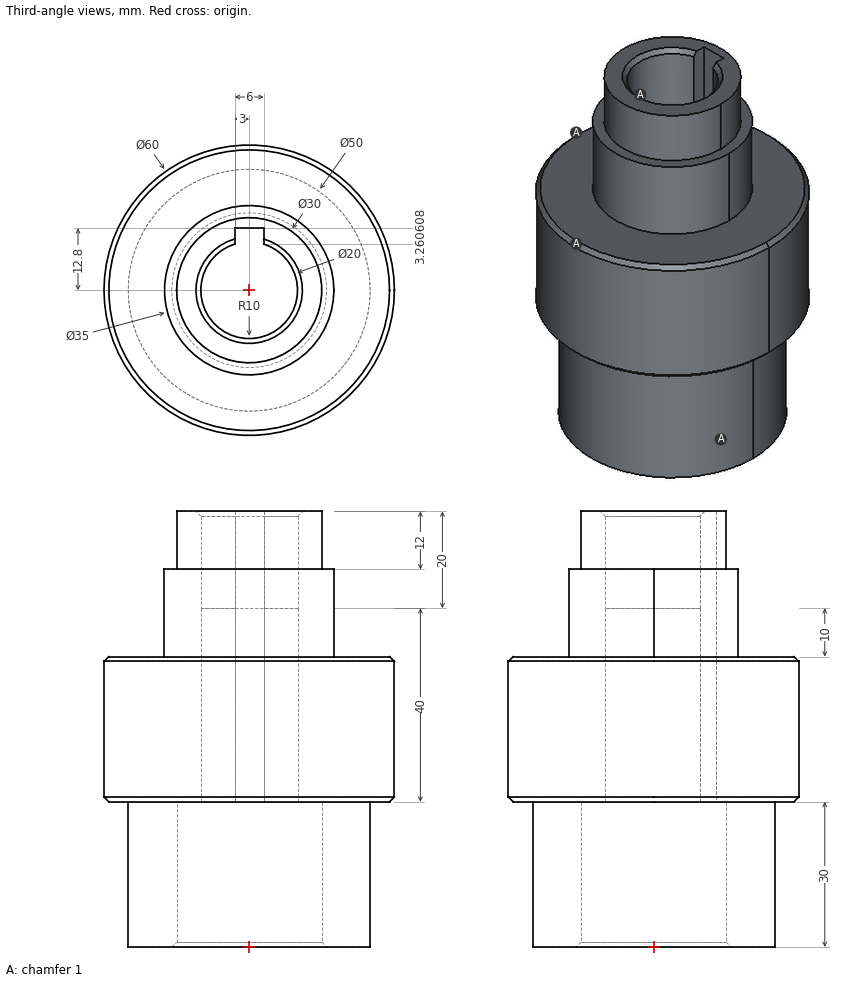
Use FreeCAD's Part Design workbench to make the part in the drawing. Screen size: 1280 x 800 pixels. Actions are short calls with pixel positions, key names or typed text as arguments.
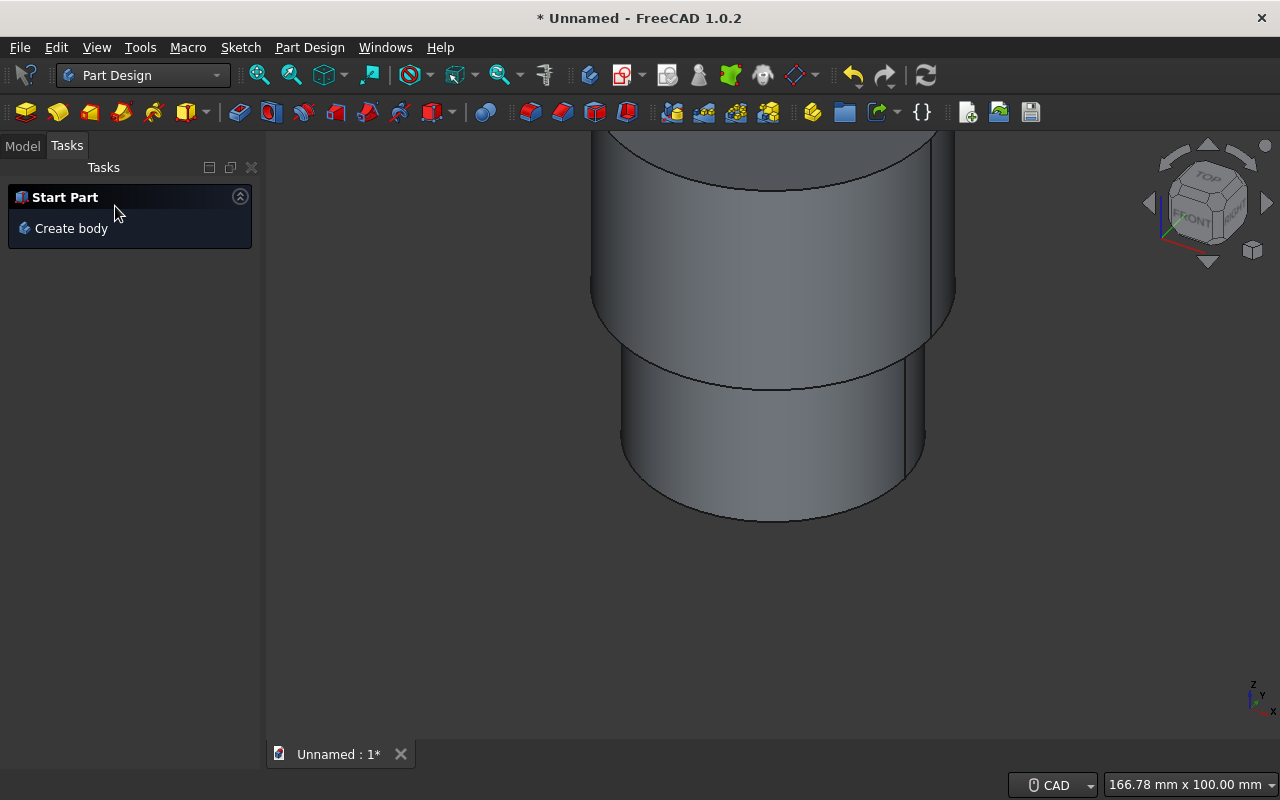
key(v)
key(f)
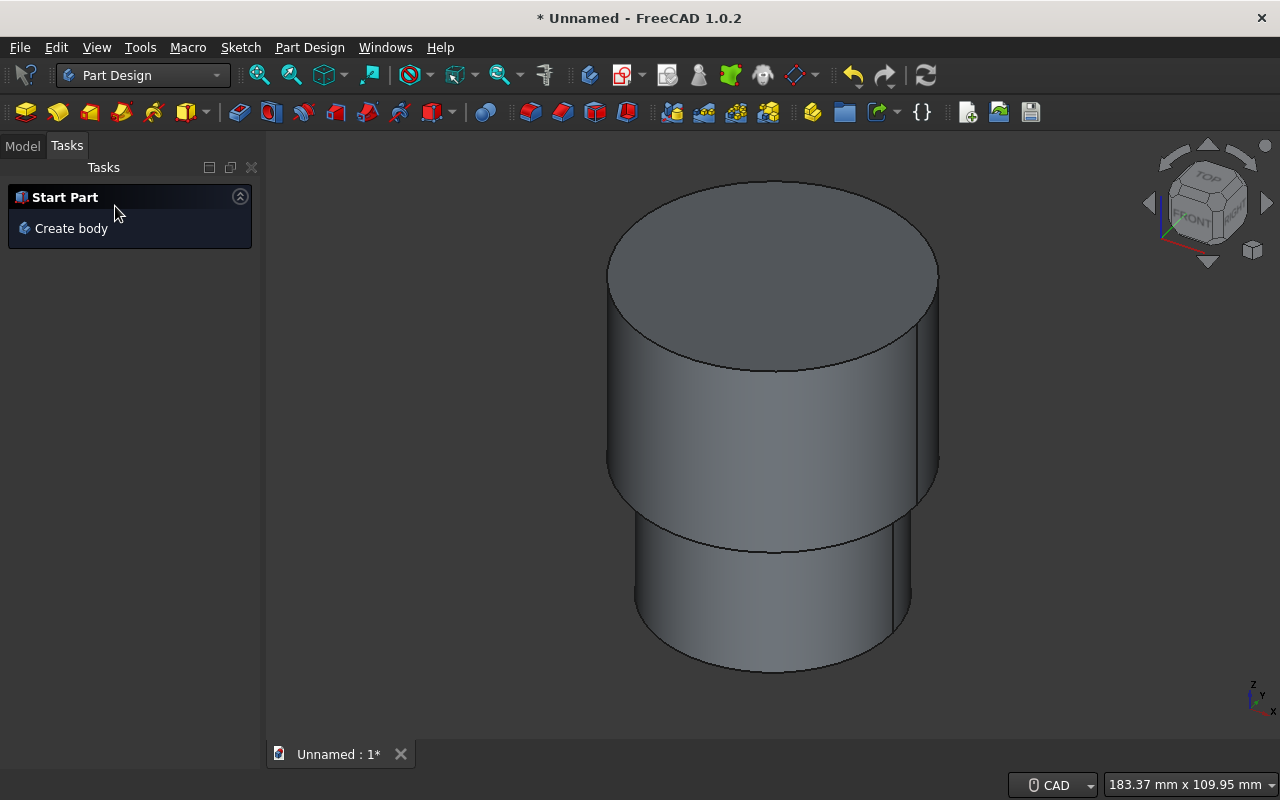
key(5)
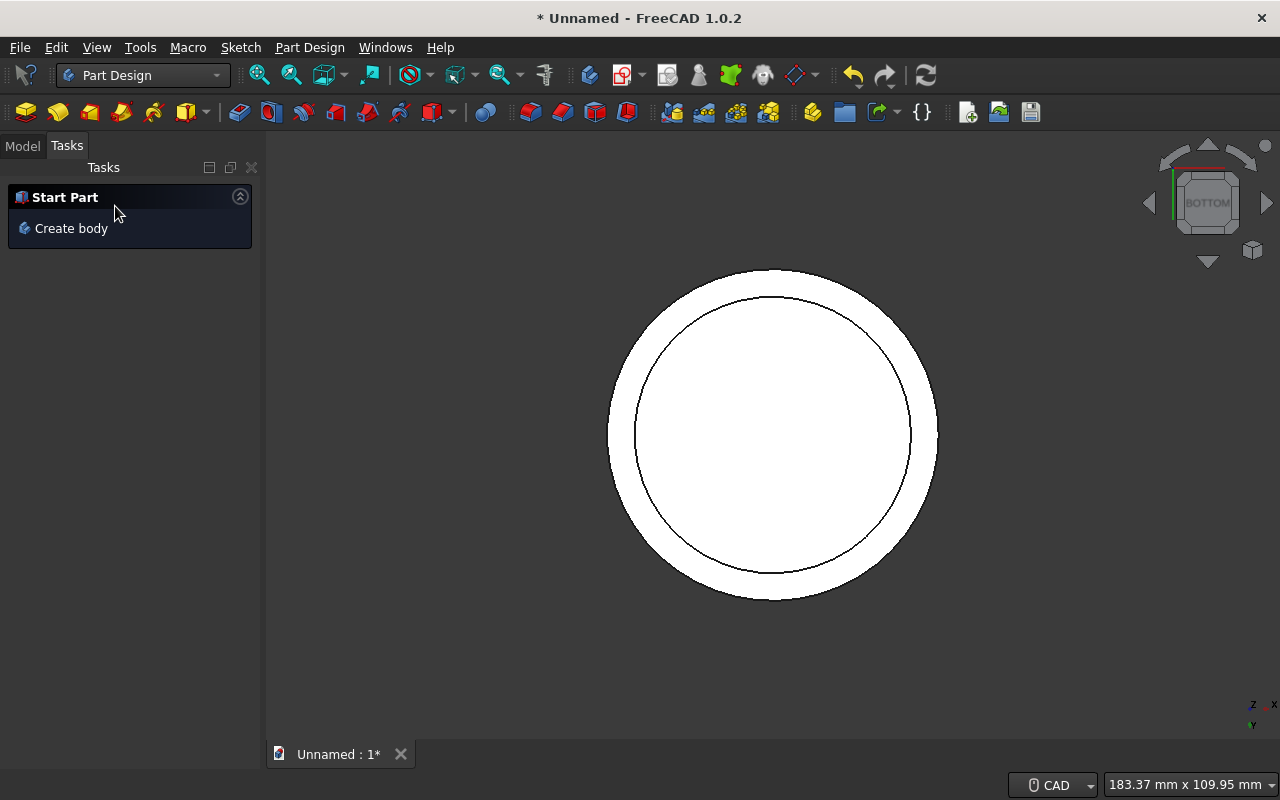
click(773, 434)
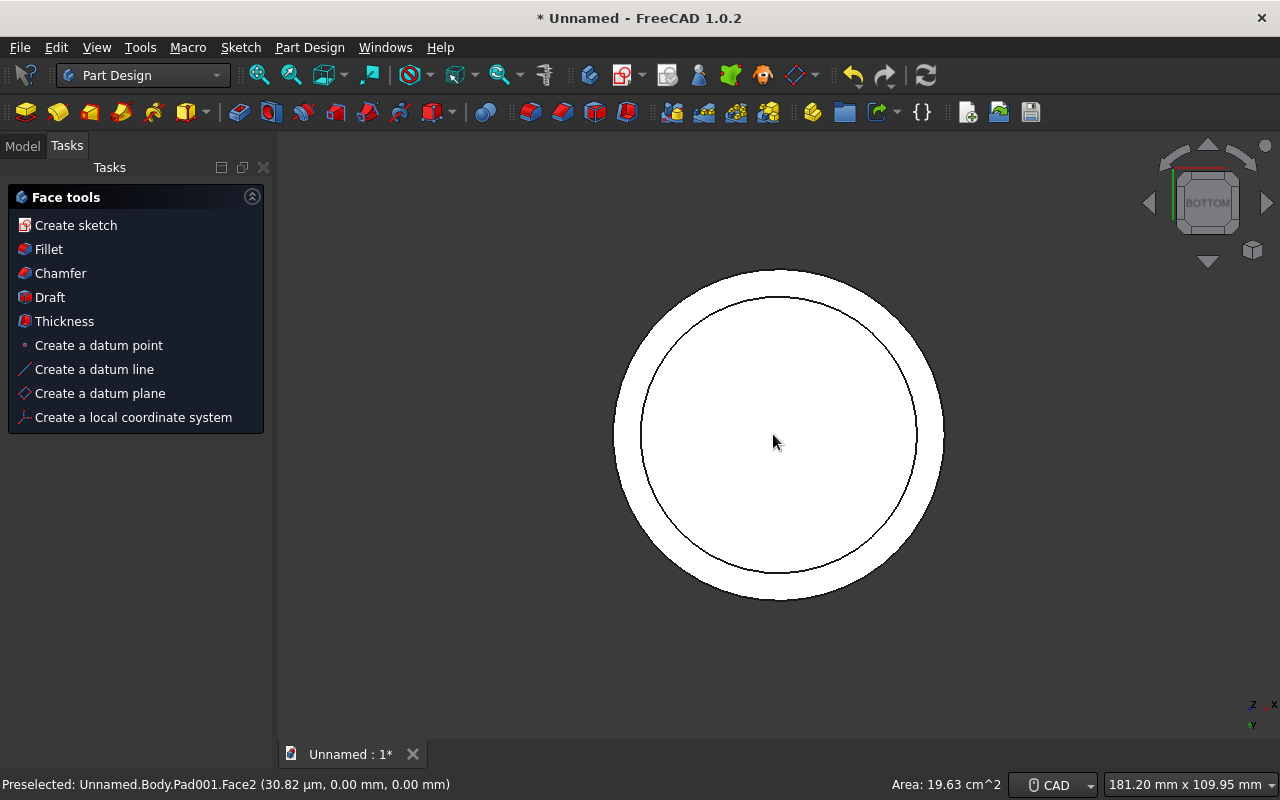
click(622, 76)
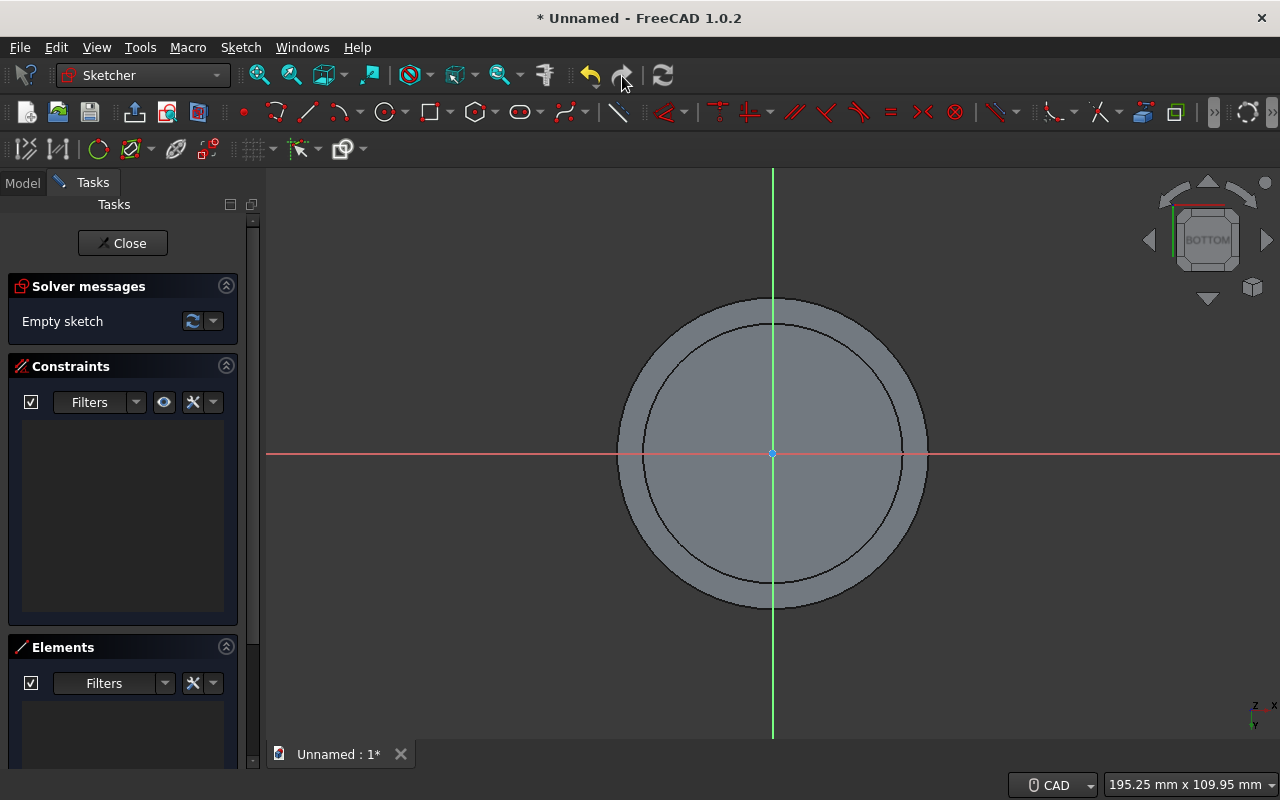
scroll(802, 454, up, 6)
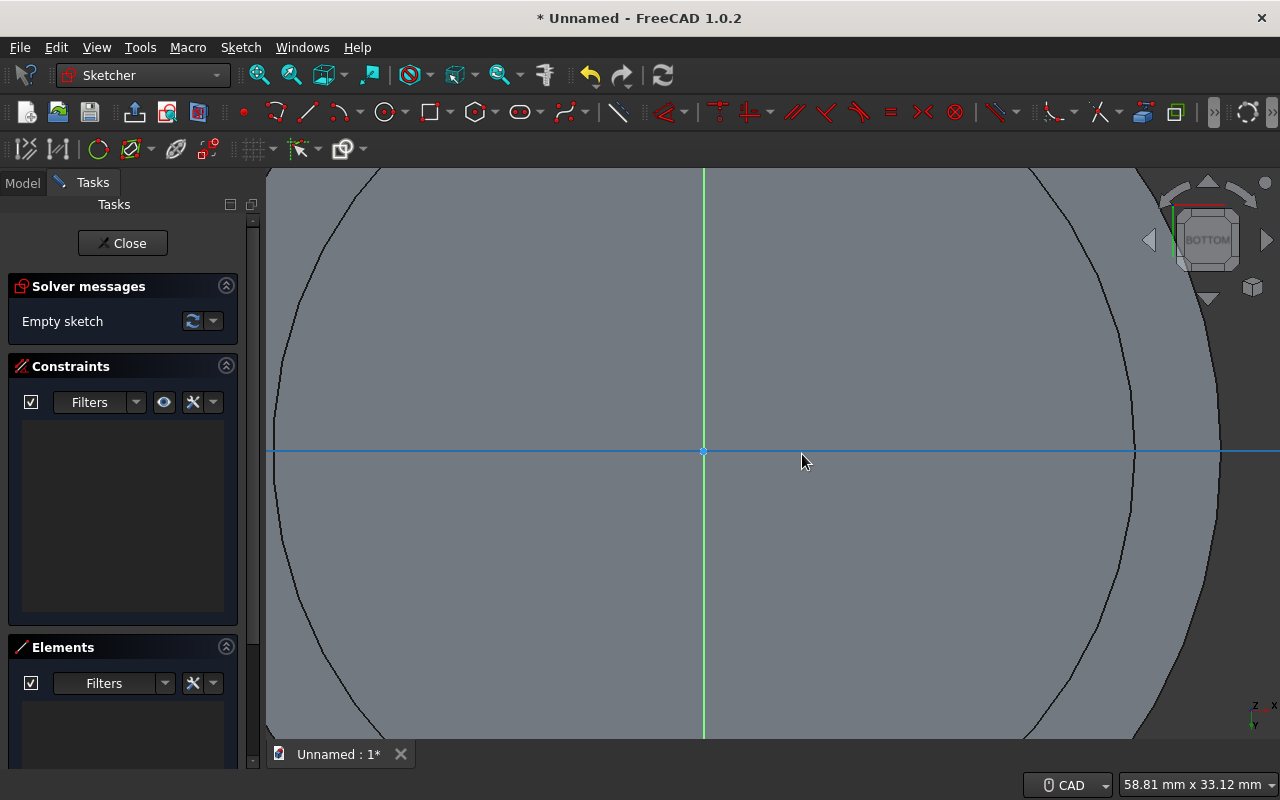
click(386, 112)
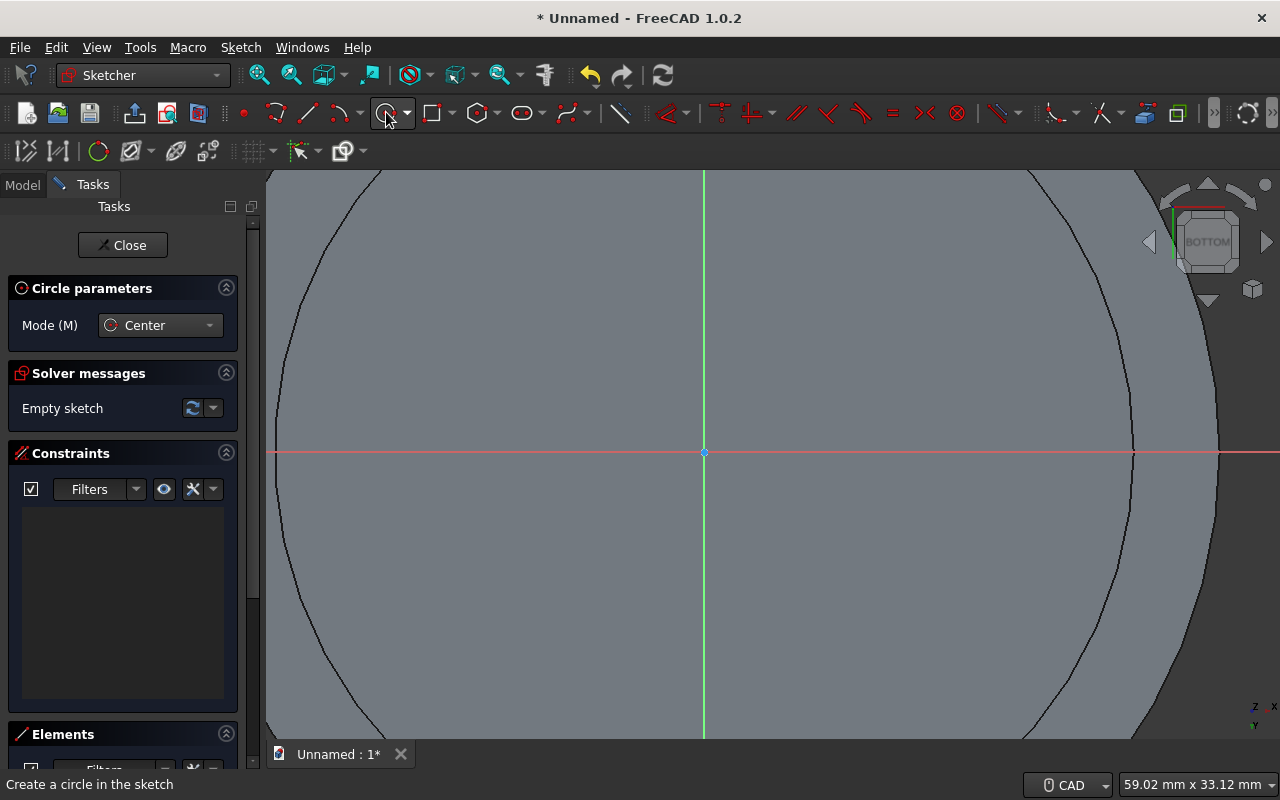
click(704, 452)
move(826, 331)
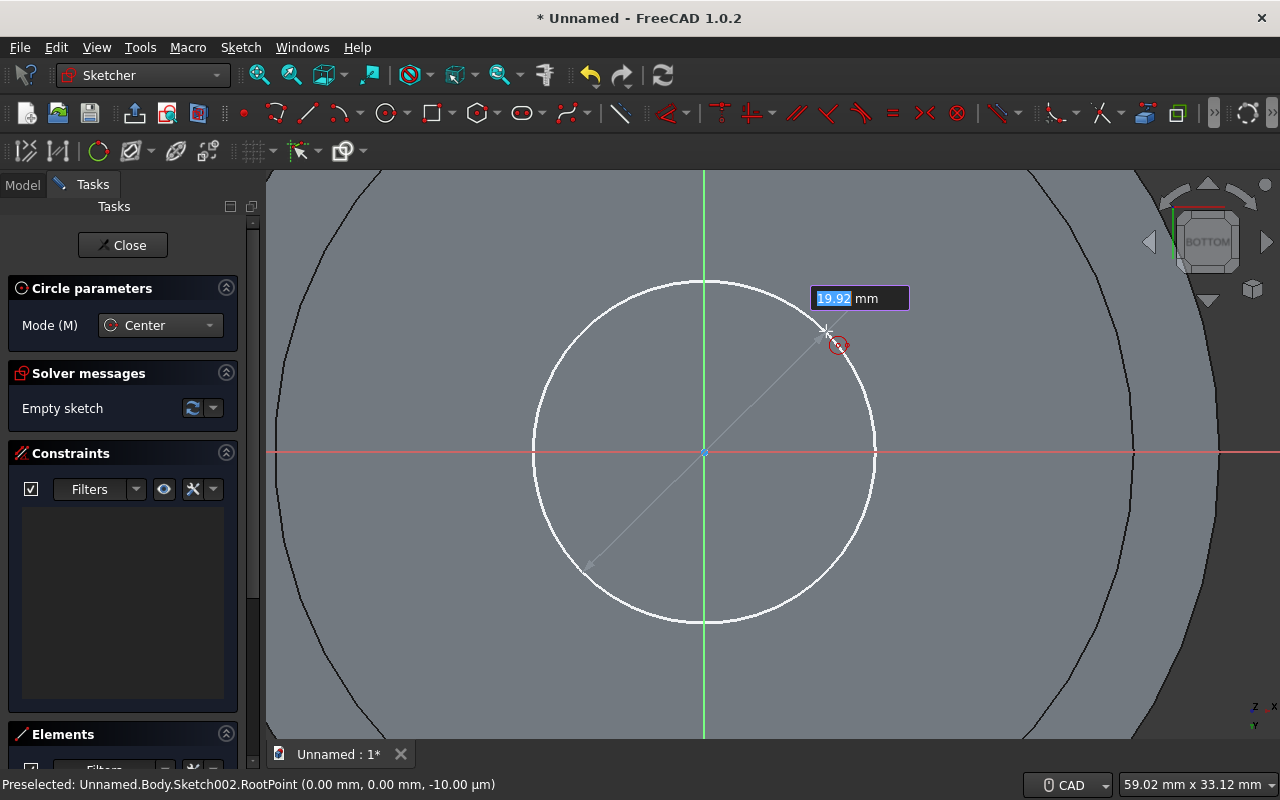
text(20)
key(Return)
key(Escape)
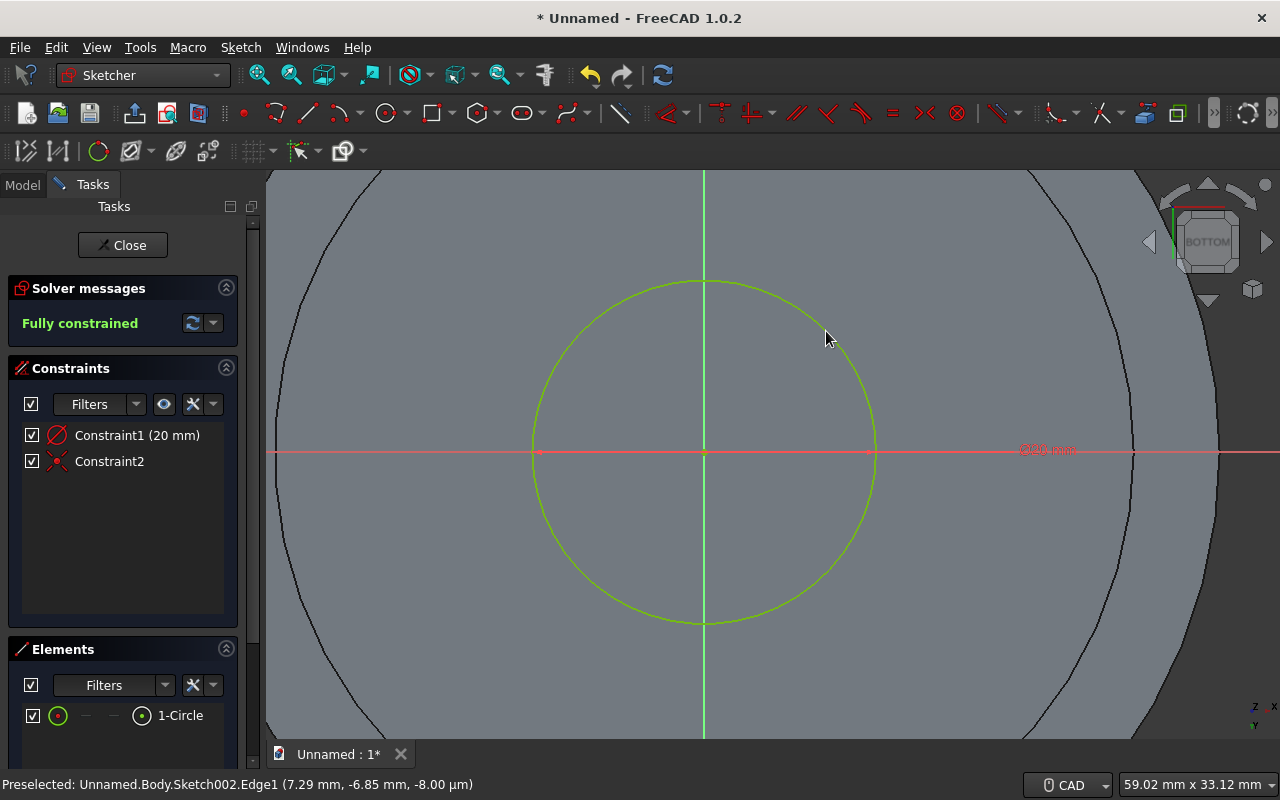
click(123, 245)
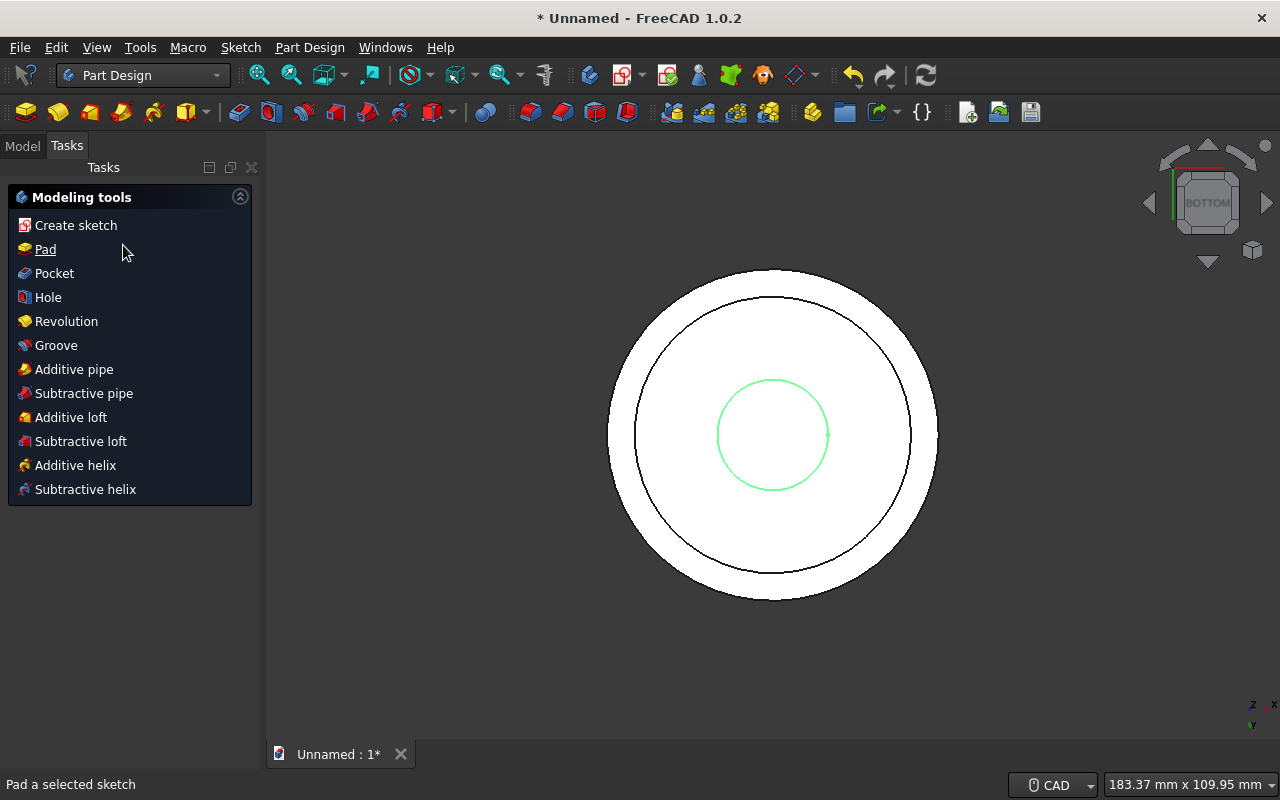
click(240, 112)